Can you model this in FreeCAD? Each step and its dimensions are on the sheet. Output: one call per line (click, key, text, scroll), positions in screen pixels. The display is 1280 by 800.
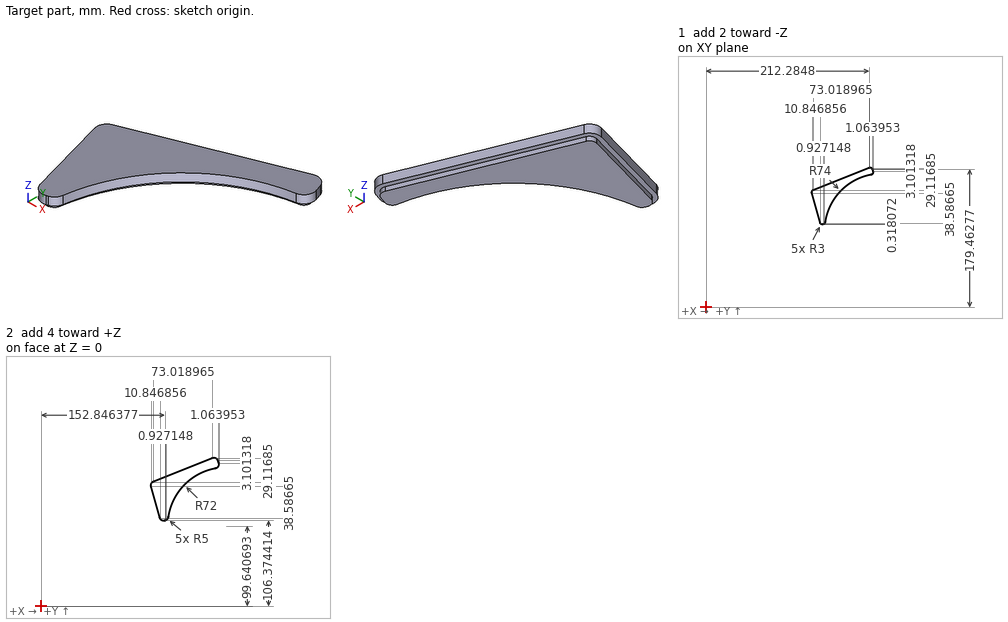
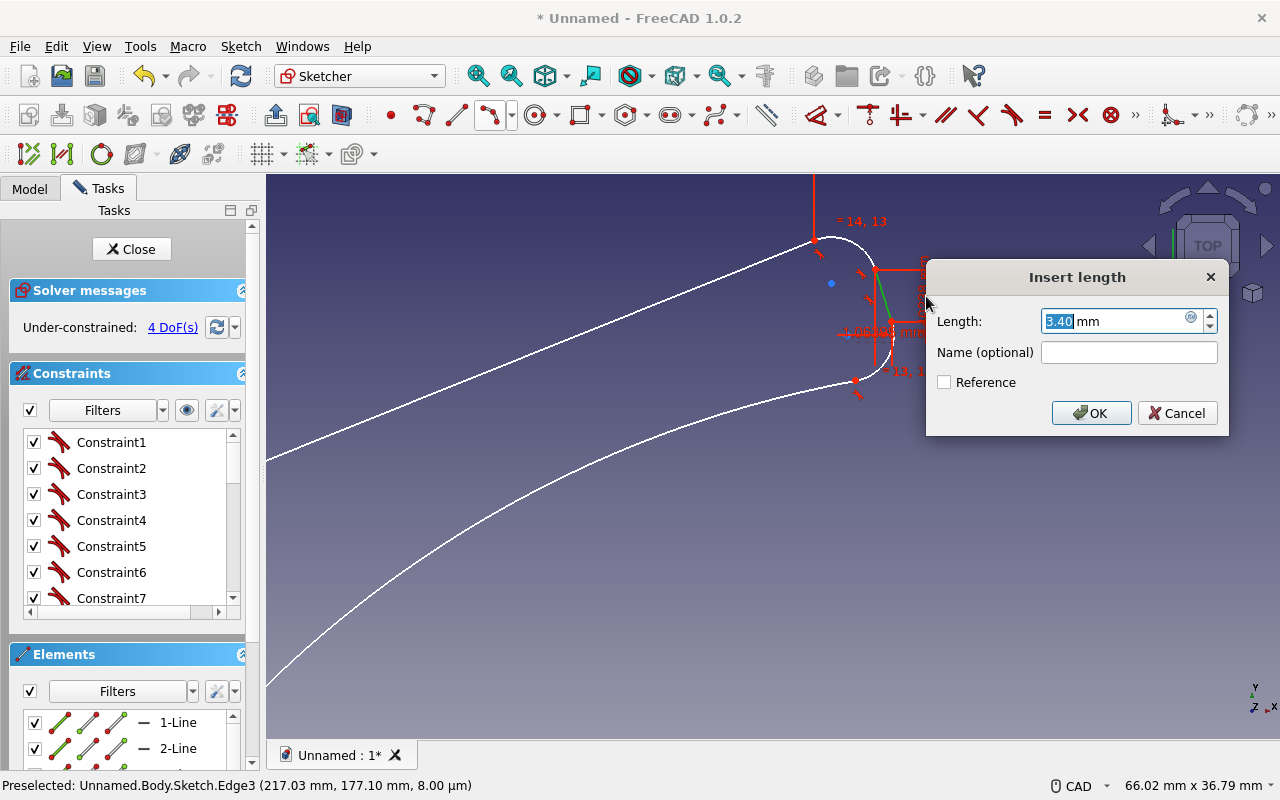
text(3.101318)
key(Return)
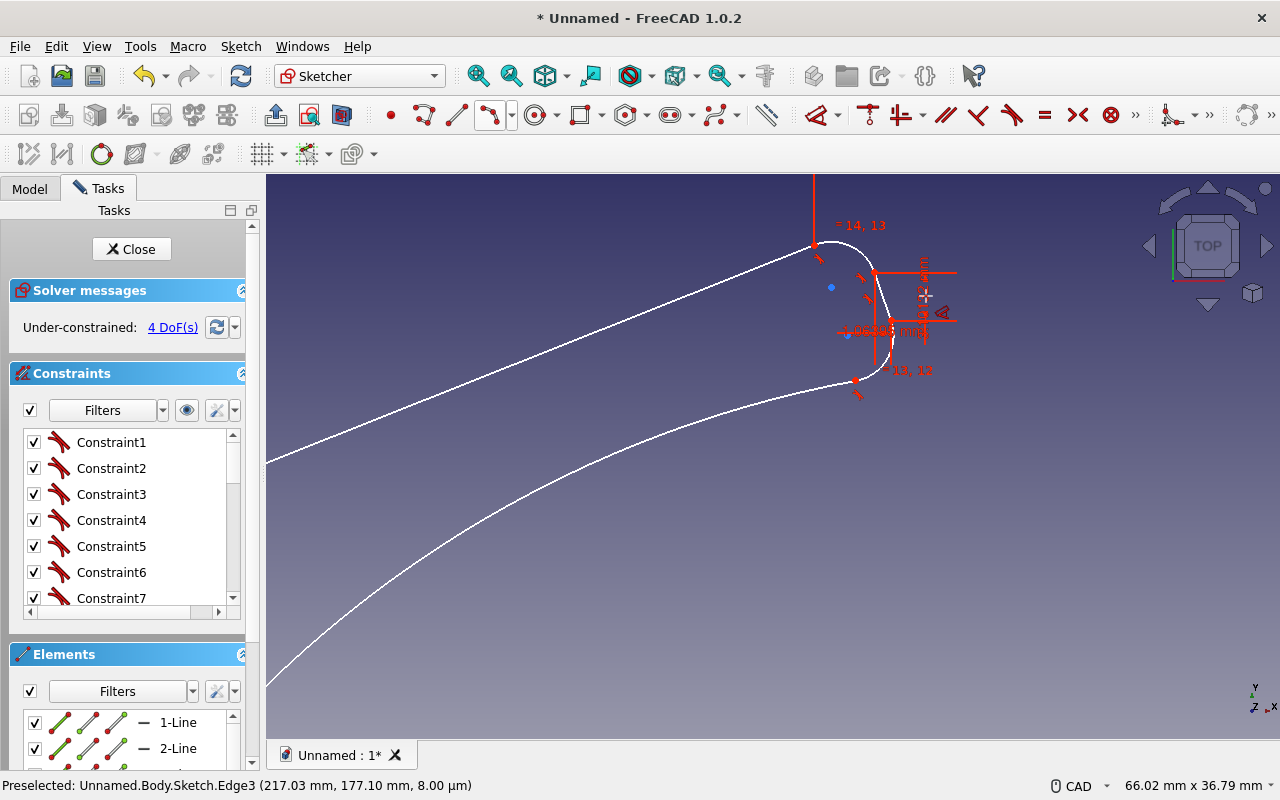
click(476, 379)
click(848, 469)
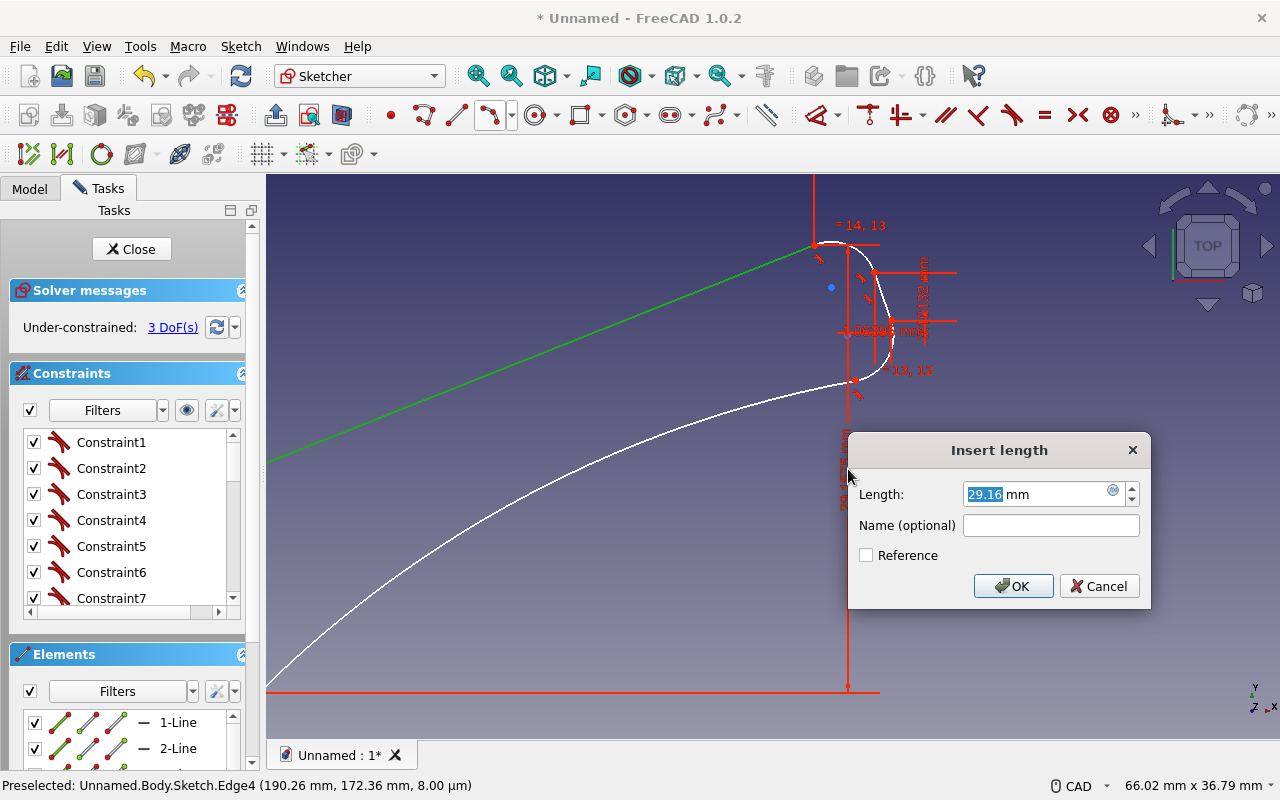
text(29.11685)
key(Return)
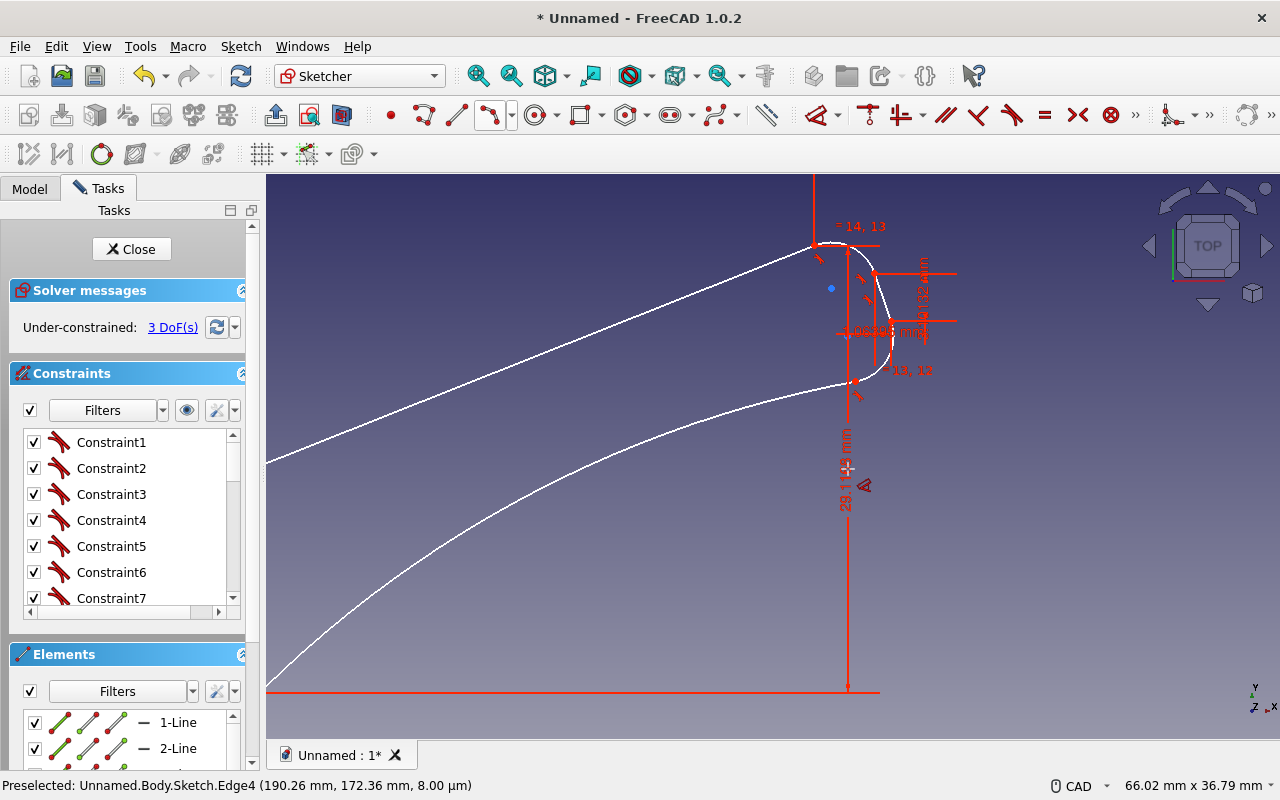
click(875, 274)
click(909, 492)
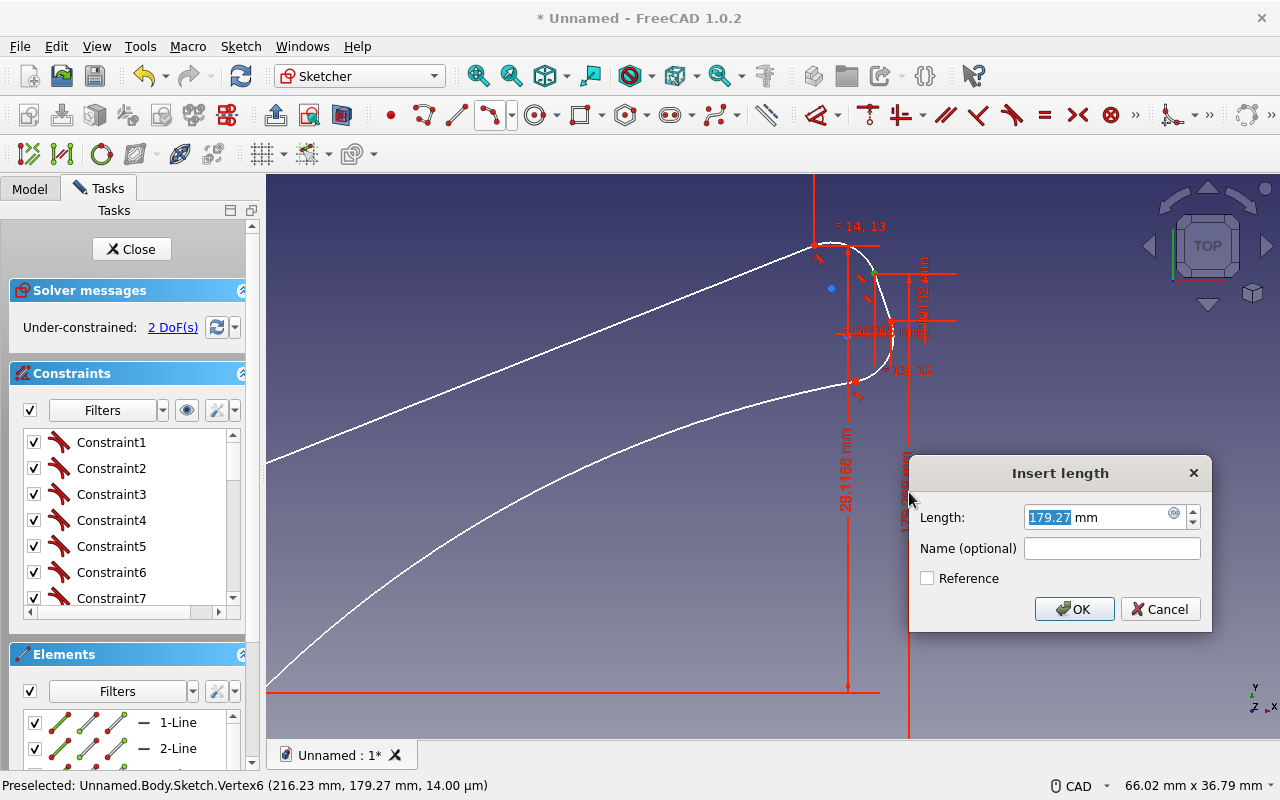
text(179.46277)
key(Return)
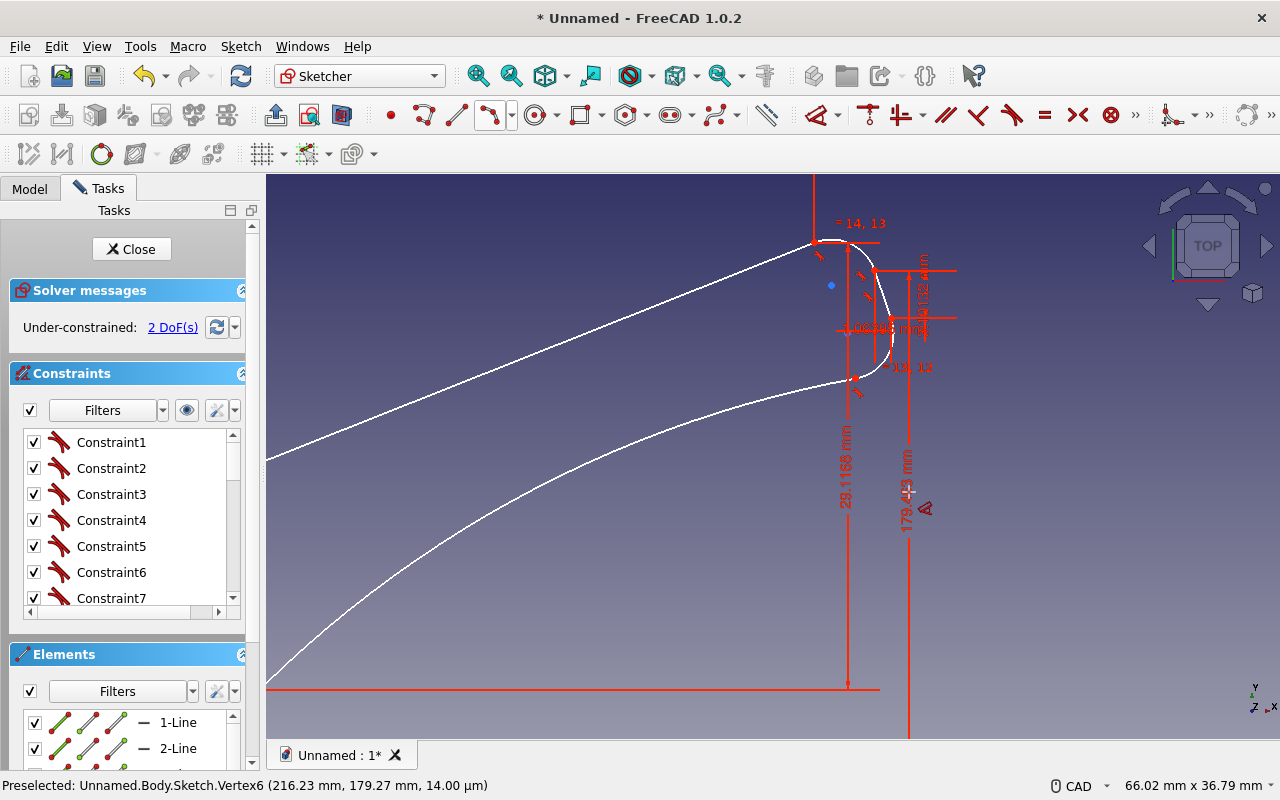
scroll(888, 306, down, 6)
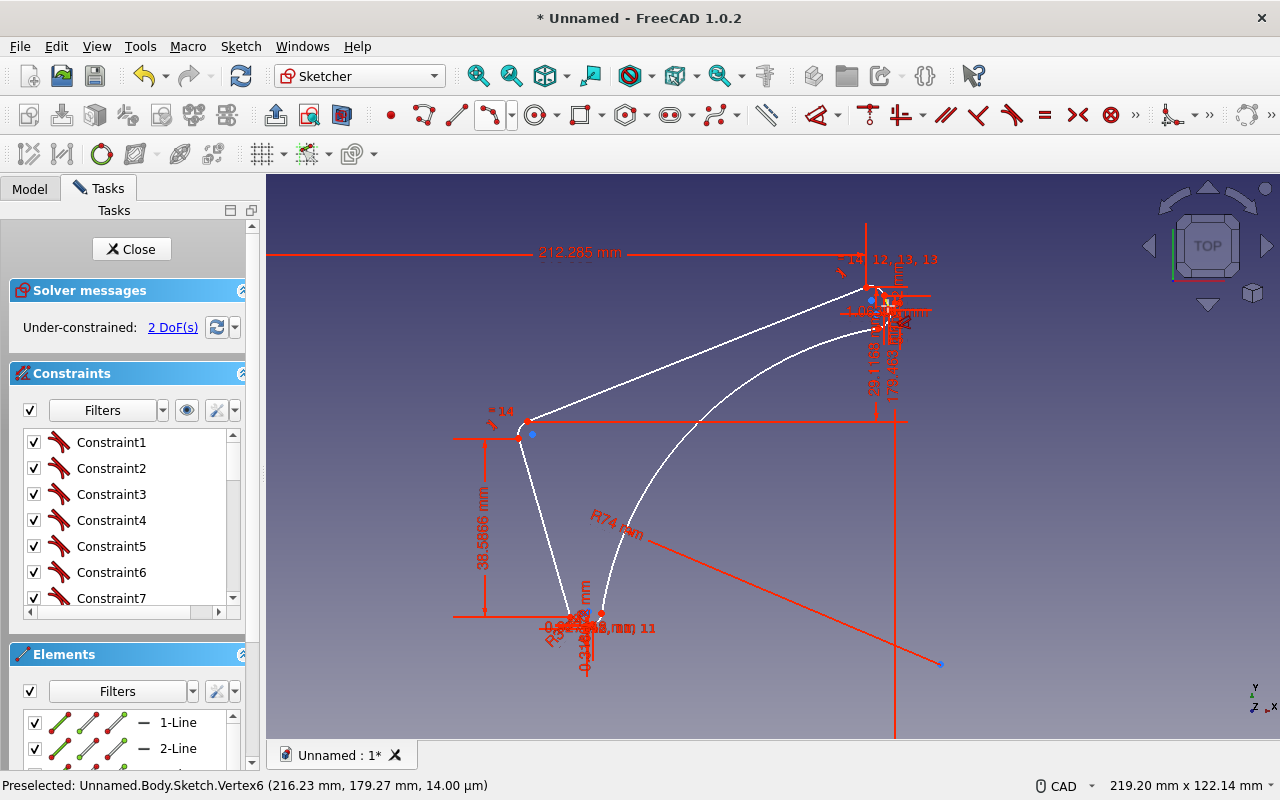
click(534, 492)
click(545, 651)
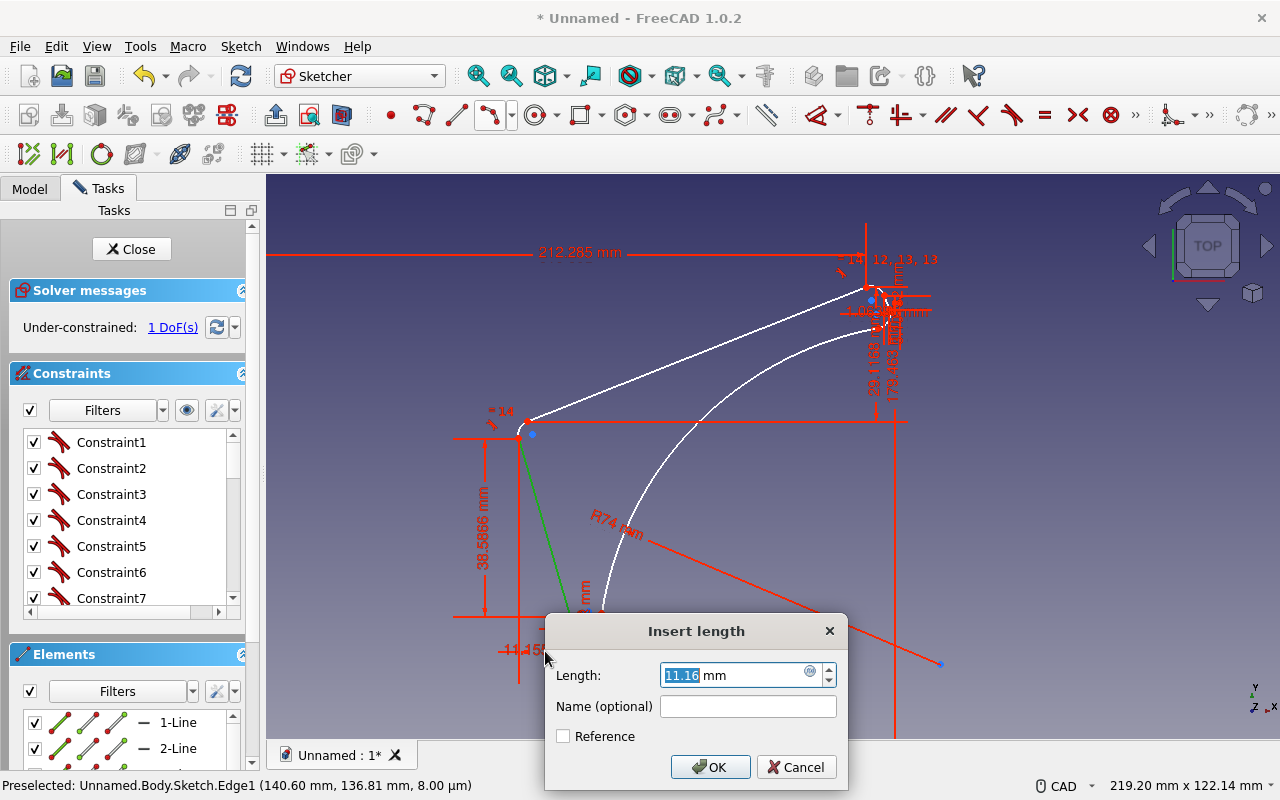
text(10.846856)
key(Return)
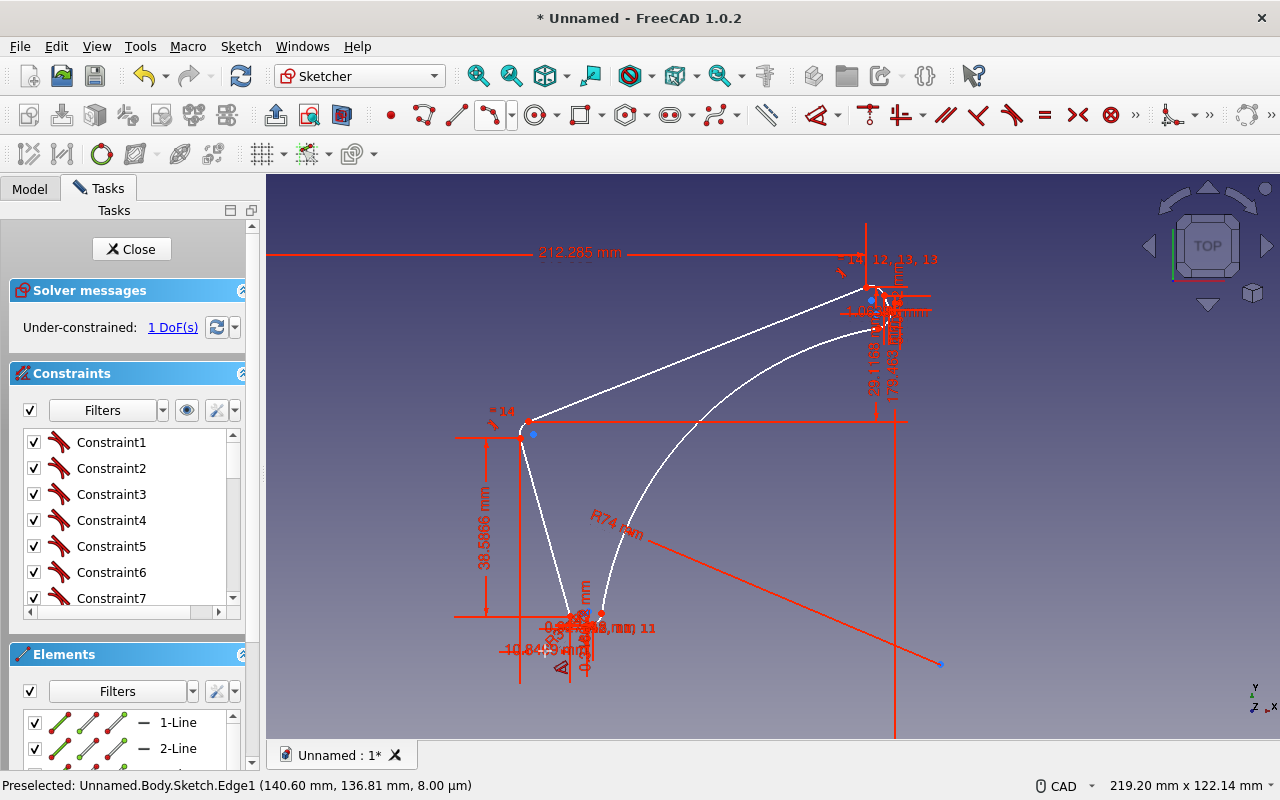
click(765, 328)
click(697, 253)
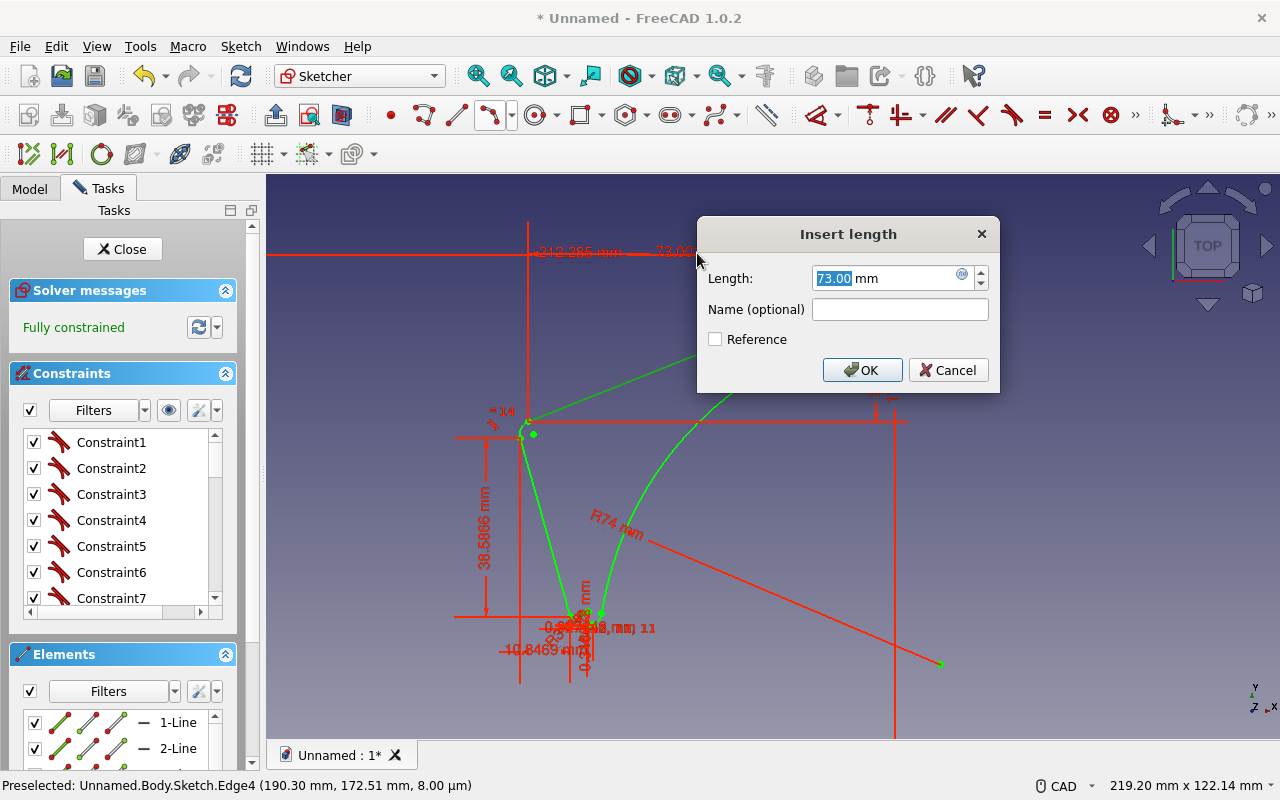
text(73.018965)
key(Return)
key(Escape)